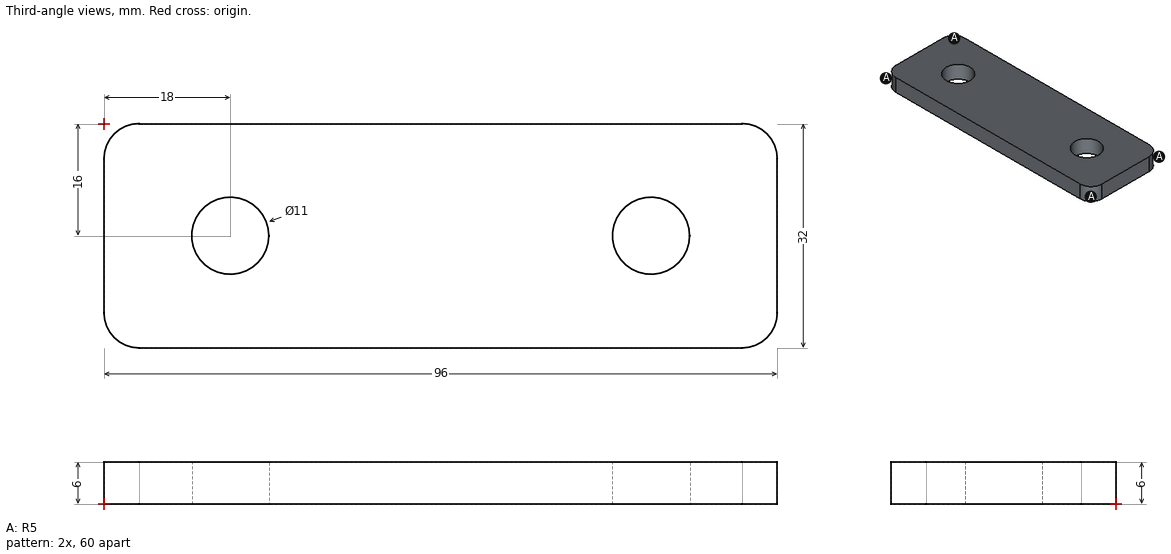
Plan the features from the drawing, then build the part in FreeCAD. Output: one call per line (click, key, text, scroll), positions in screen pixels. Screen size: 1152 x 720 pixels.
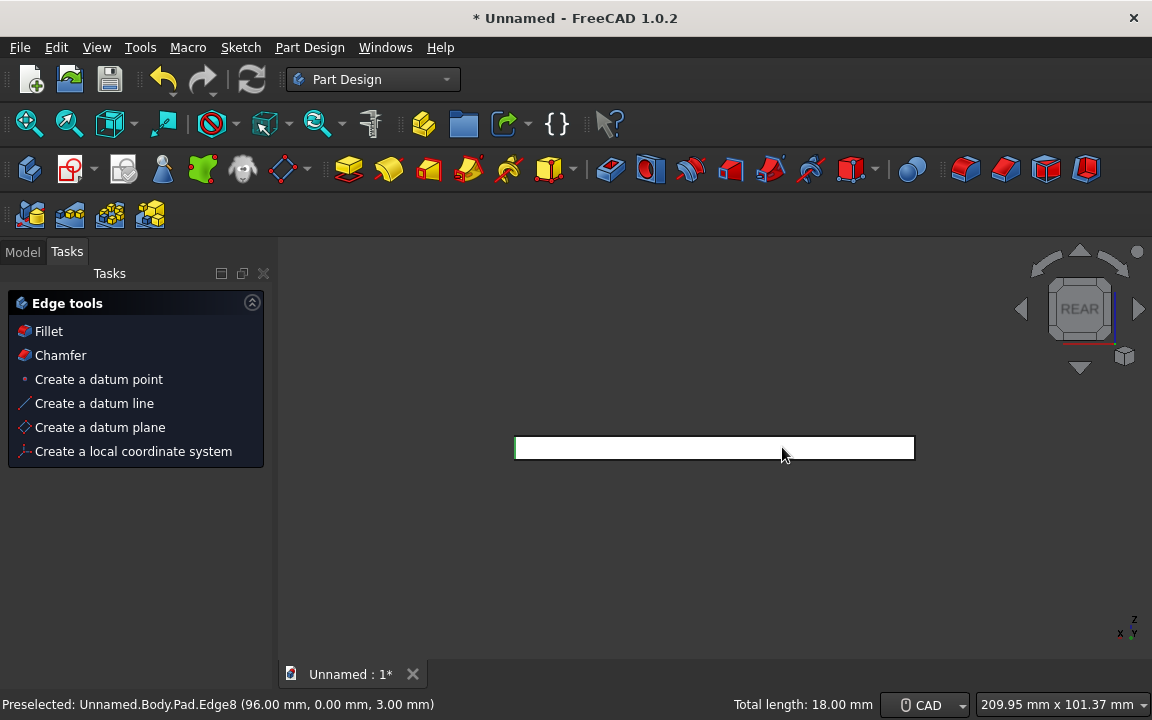
click(915, 447, ctrl)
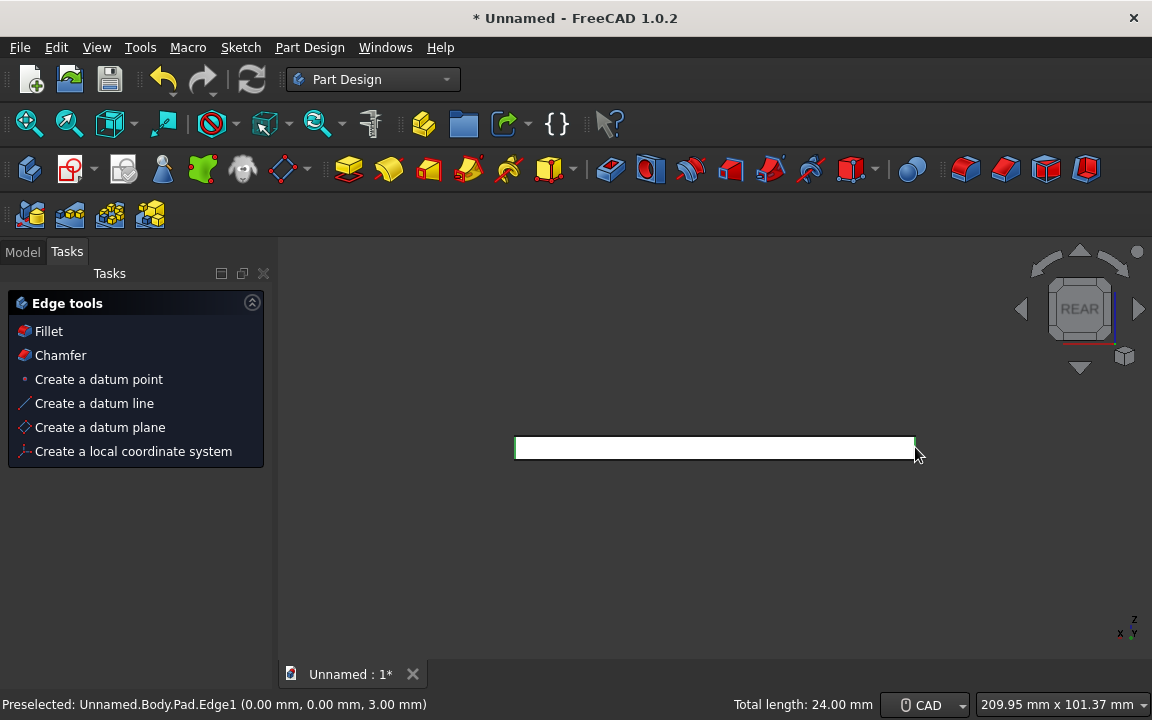
click(966, 170)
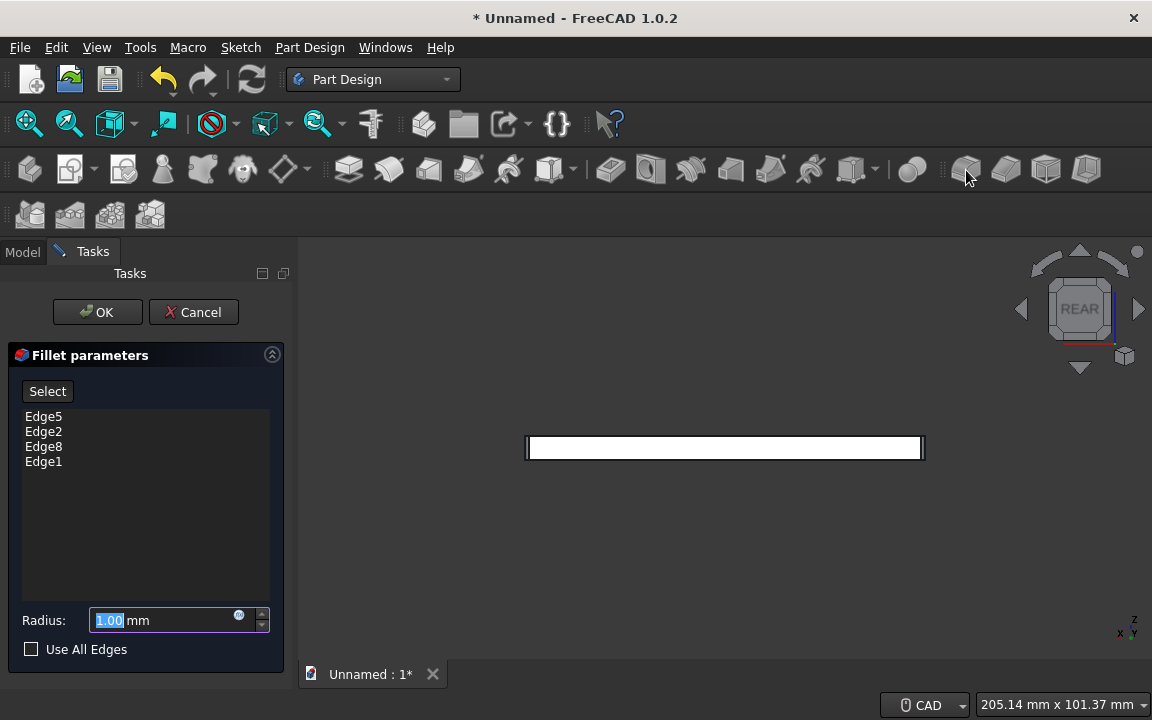
text(5)
key(Tab)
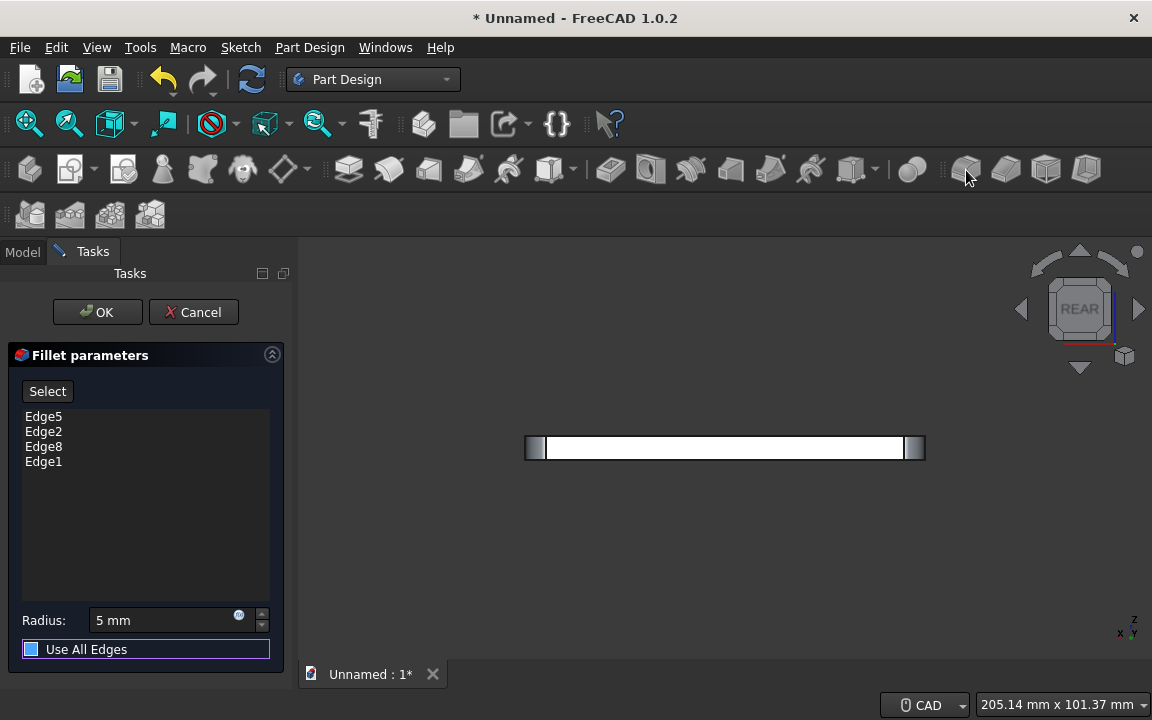
click(98, 312)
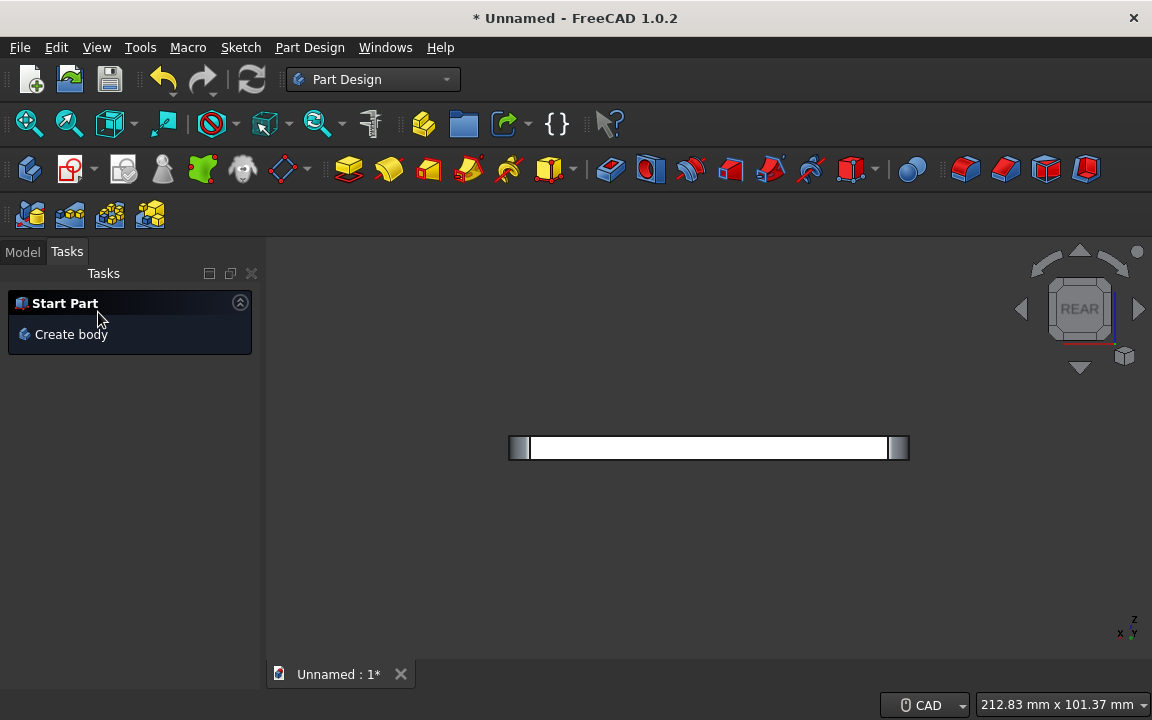
key(0)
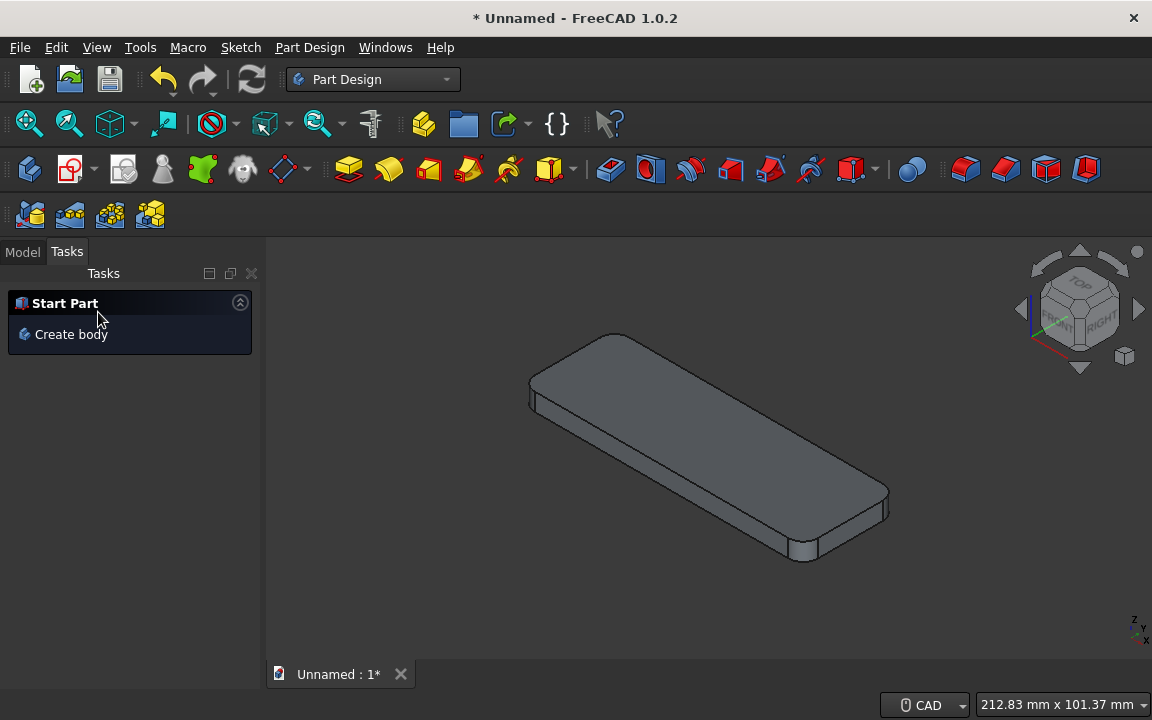
click(790, 483)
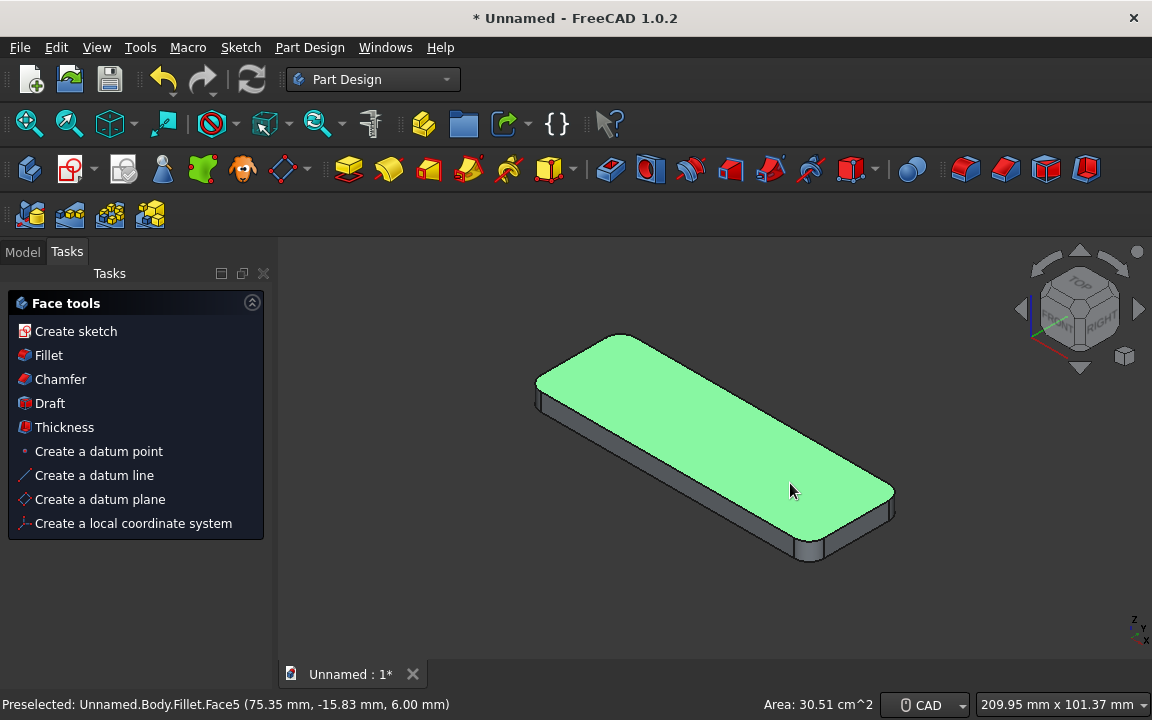
click(70, 170)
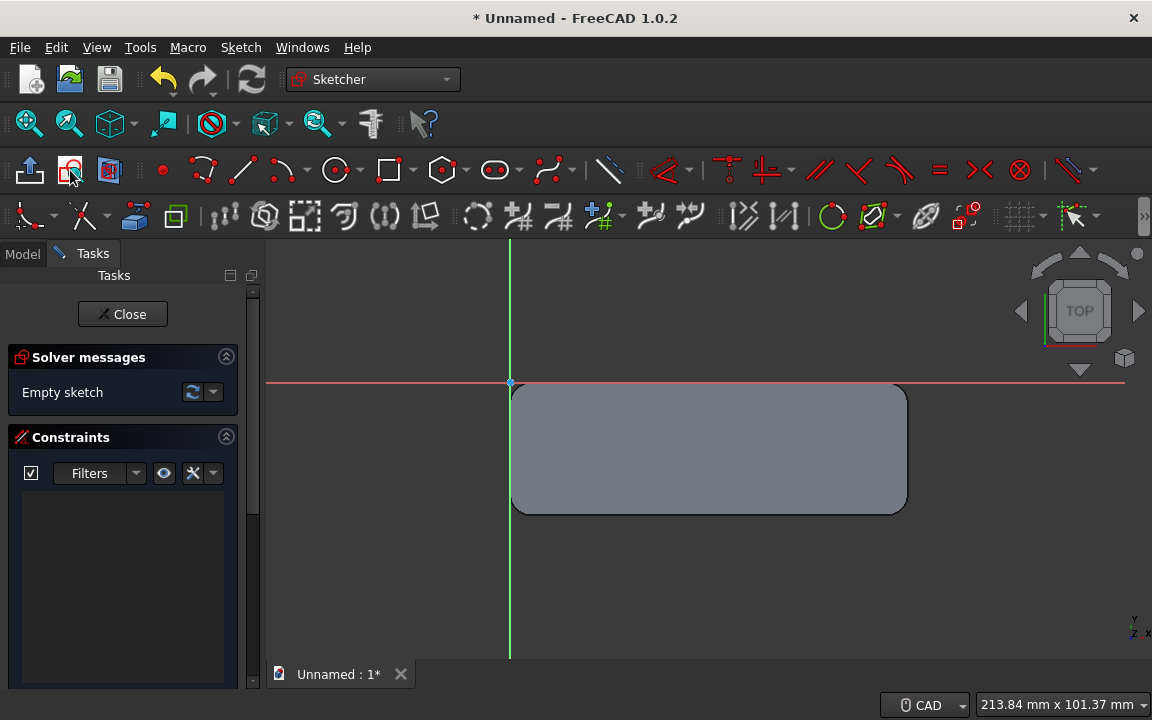
scroll(511, 415, up, 5)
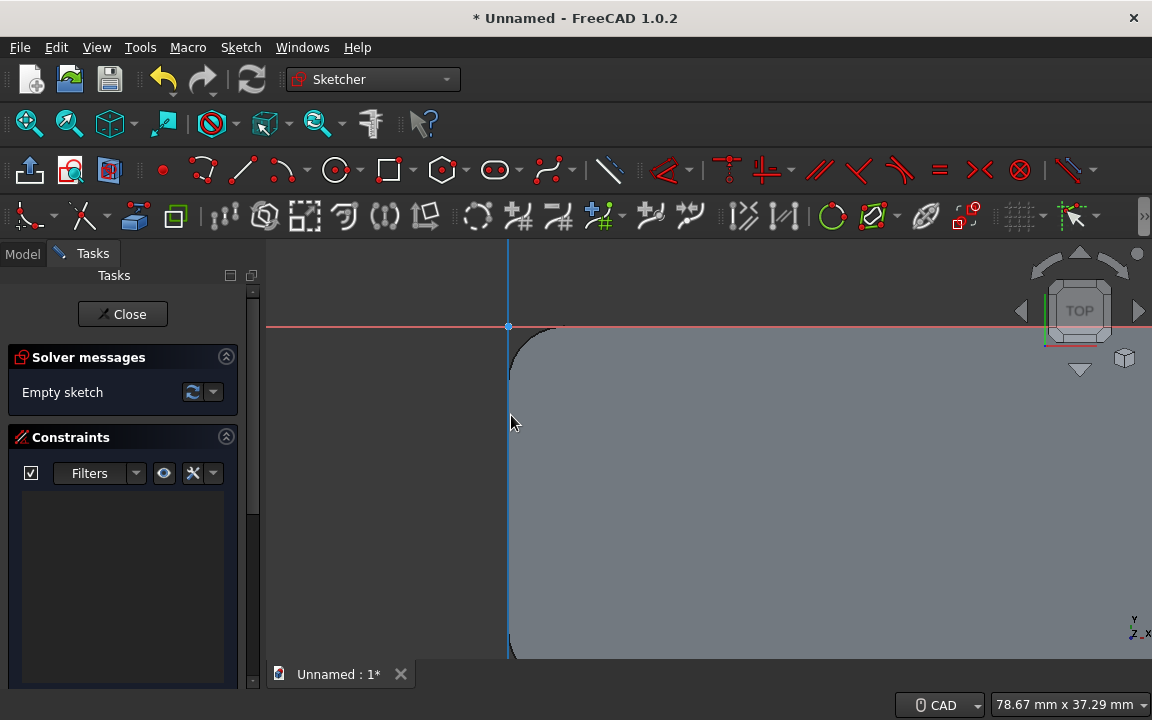
click(336, 170)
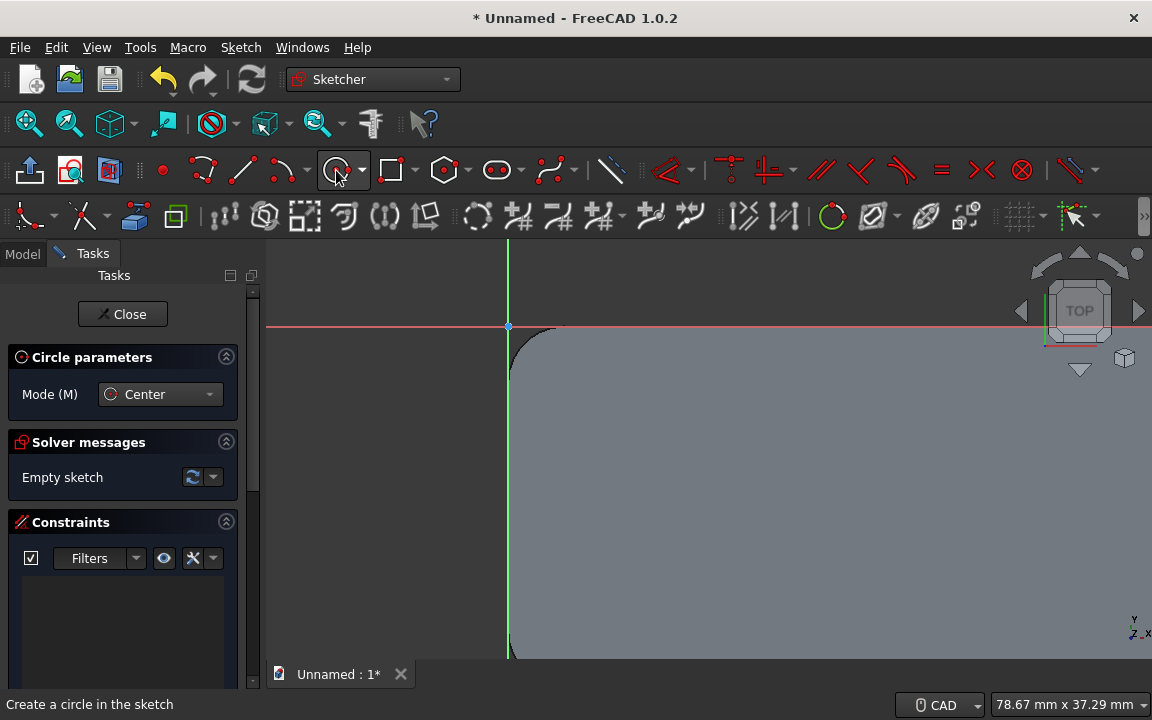
click(711, 507)
move(755, 463)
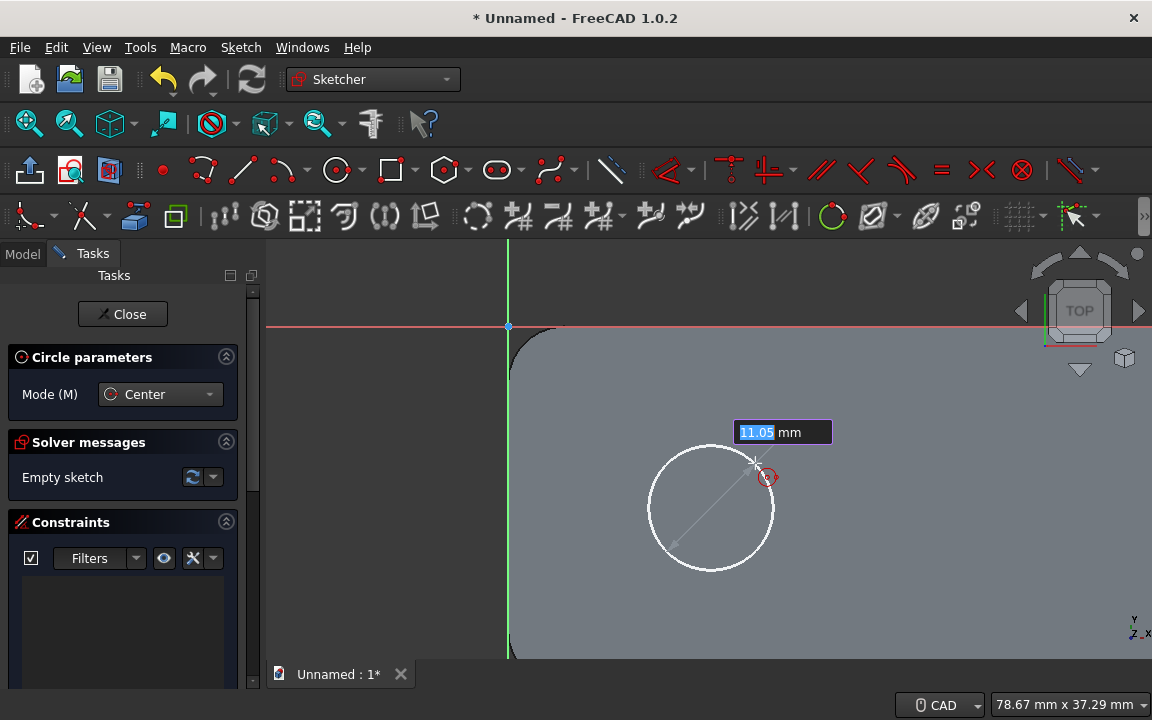
text(11)
key(Return)
key(Escape)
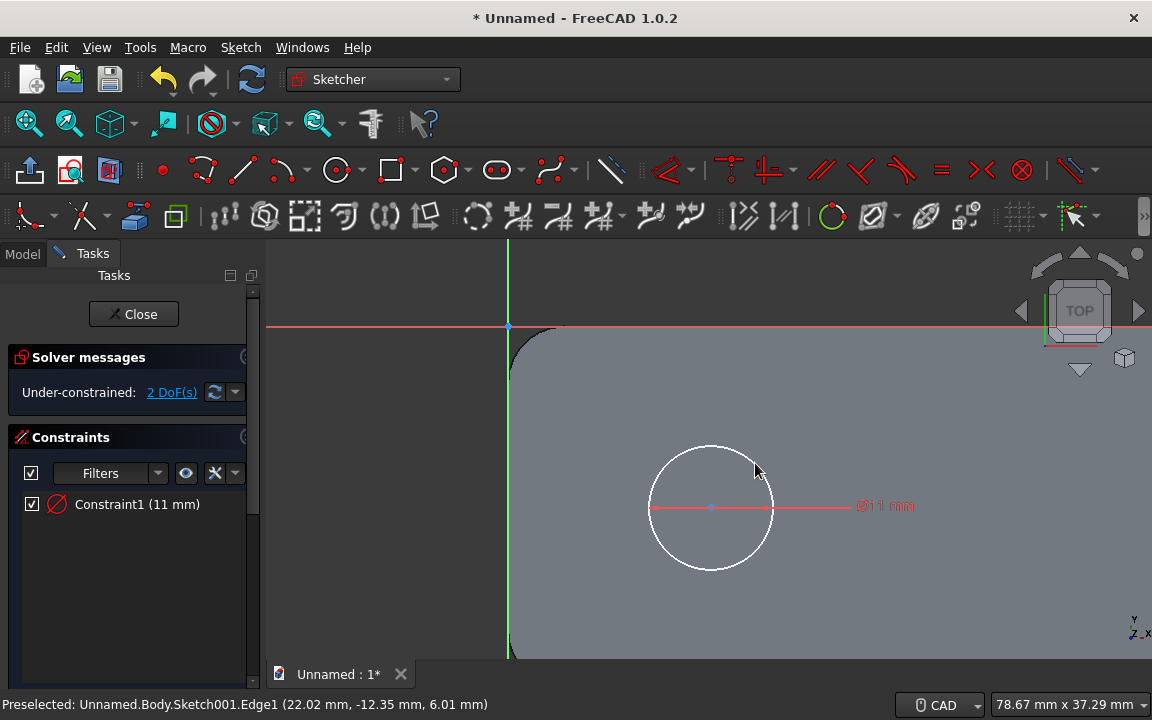
click(711, 508)